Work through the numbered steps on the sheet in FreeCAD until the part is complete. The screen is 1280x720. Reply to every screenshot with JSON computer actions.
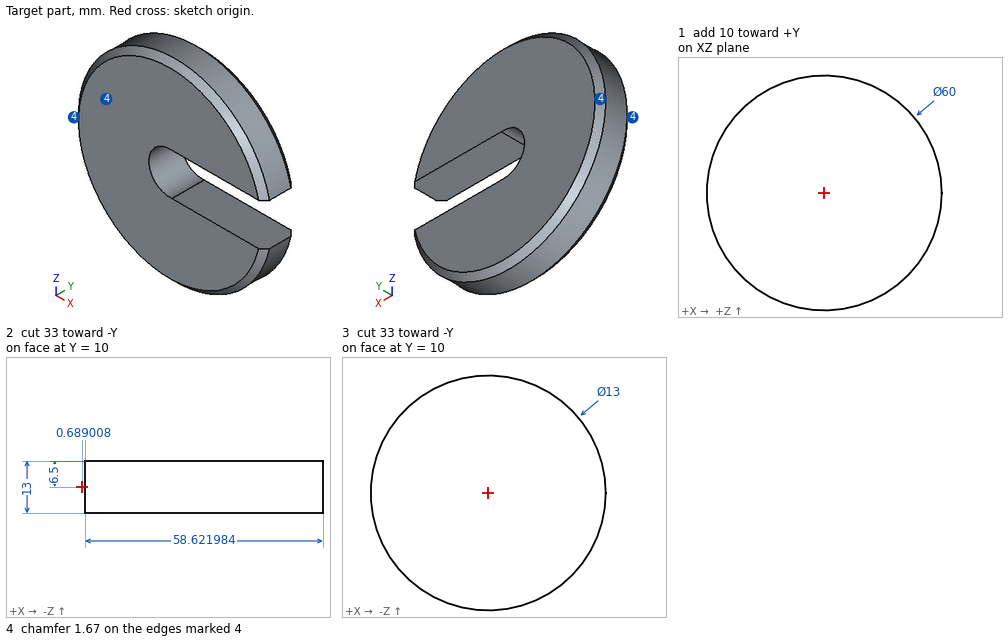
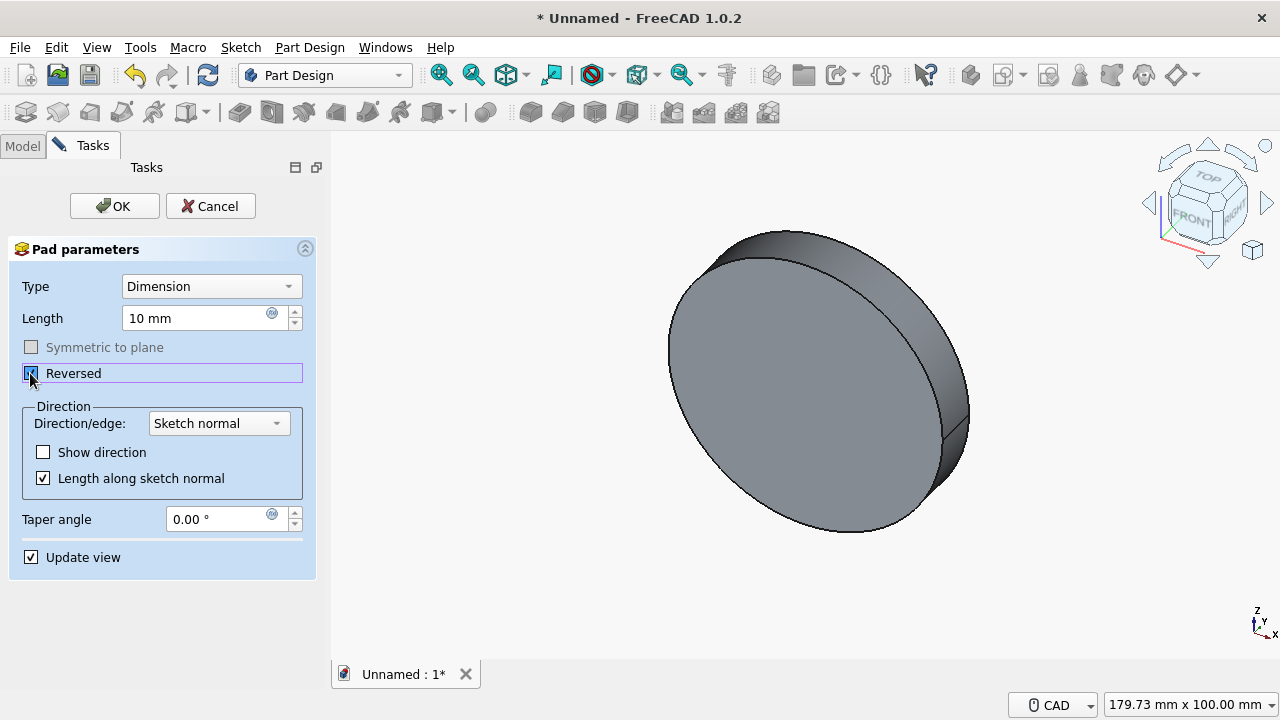
{"action": "left_click", "coordinate": [115, 206]}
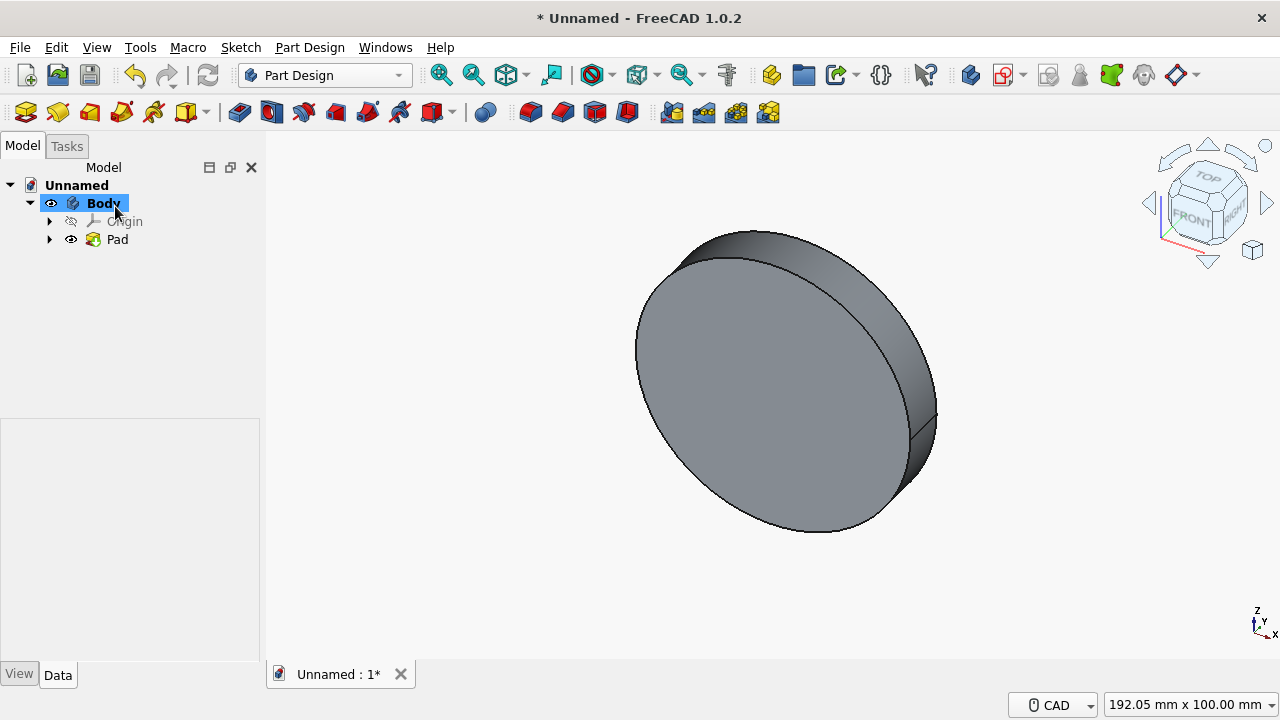
{"action": "key", "text": "4"}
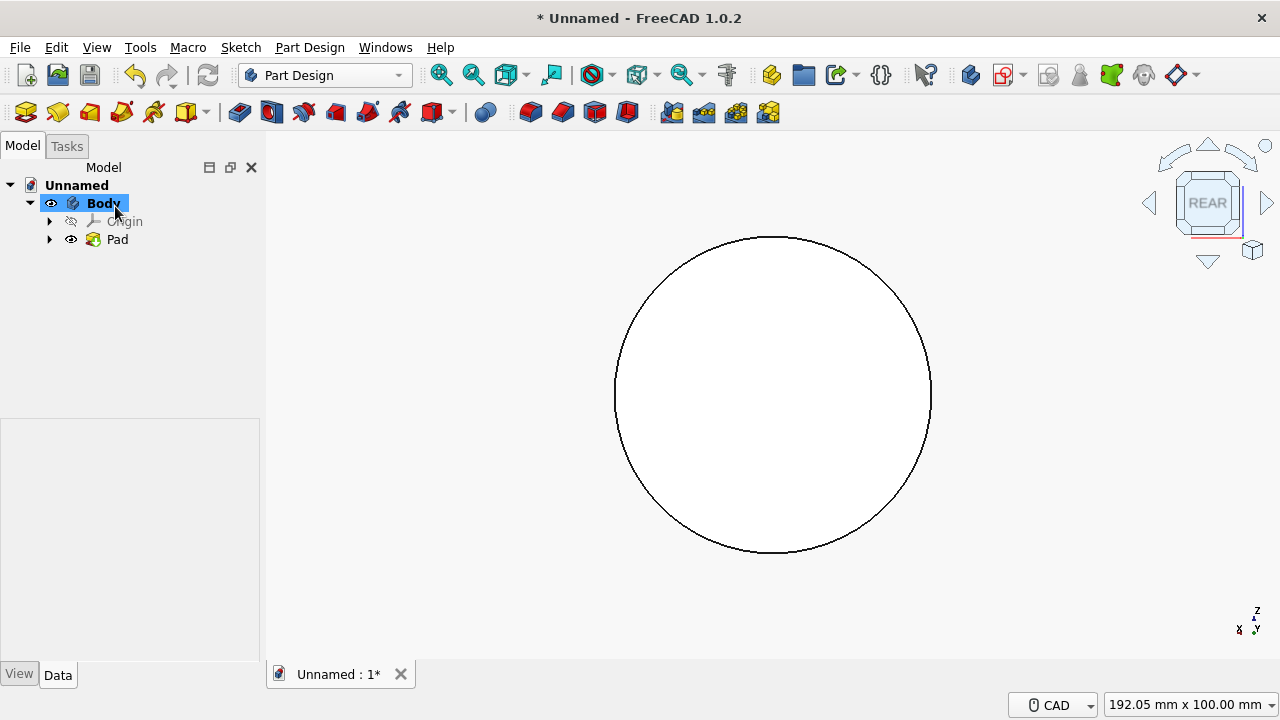
{"action": "left_click", "coordinate": [773, 394]}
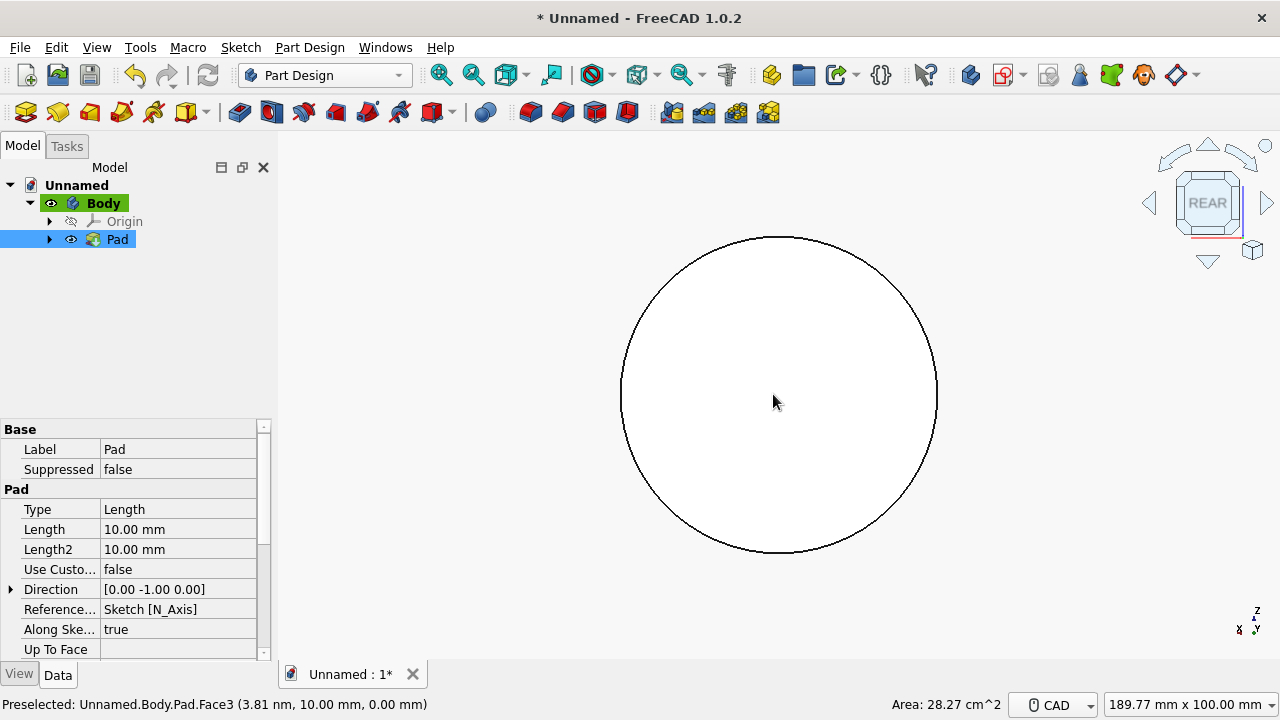
{"action": "left_click", "coordinate": [1004, 76]}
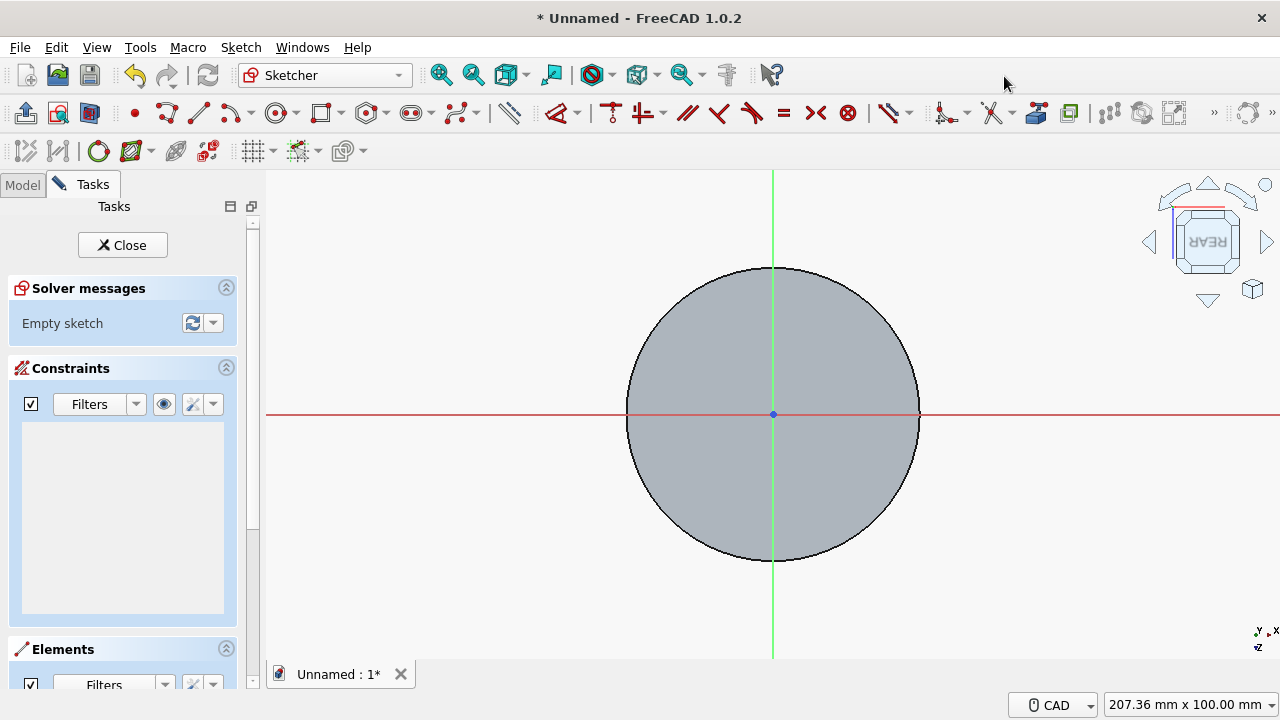
{"action": "scroll", "coordinate": [1115, 415], "scroll_direction": "up", "scroll_amount": 3}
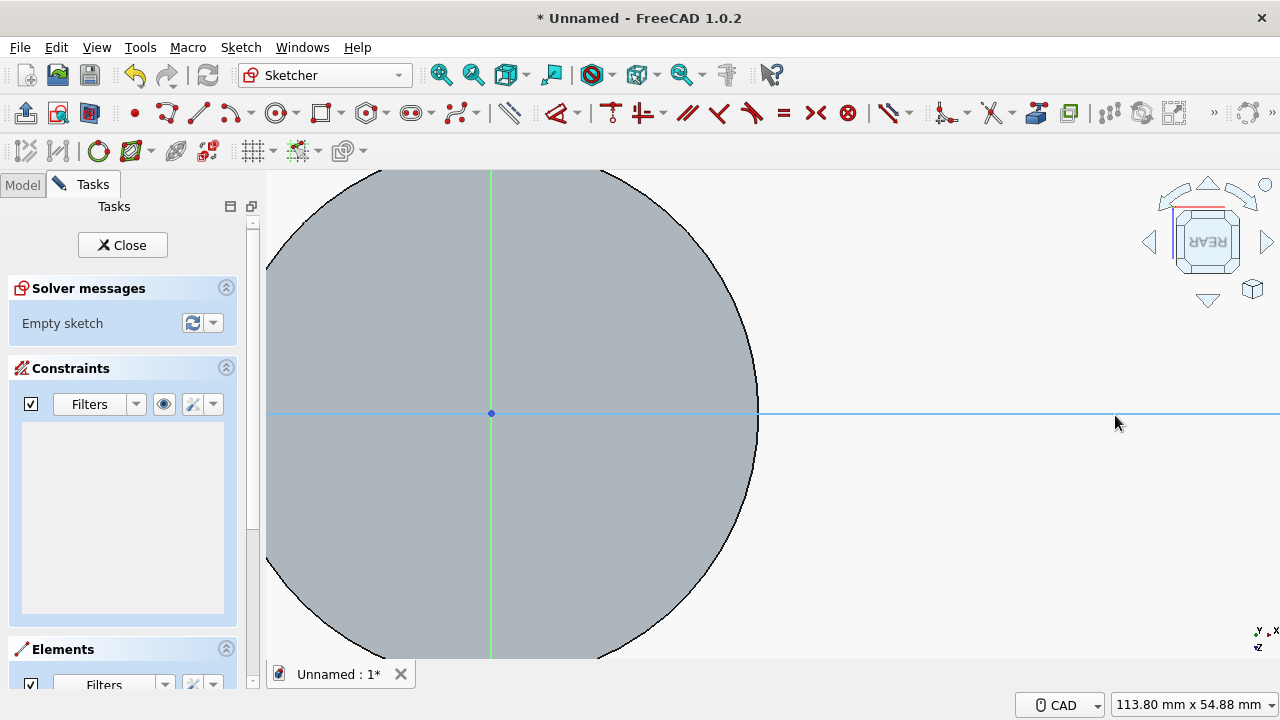
{"action": "key", "text": "g r"}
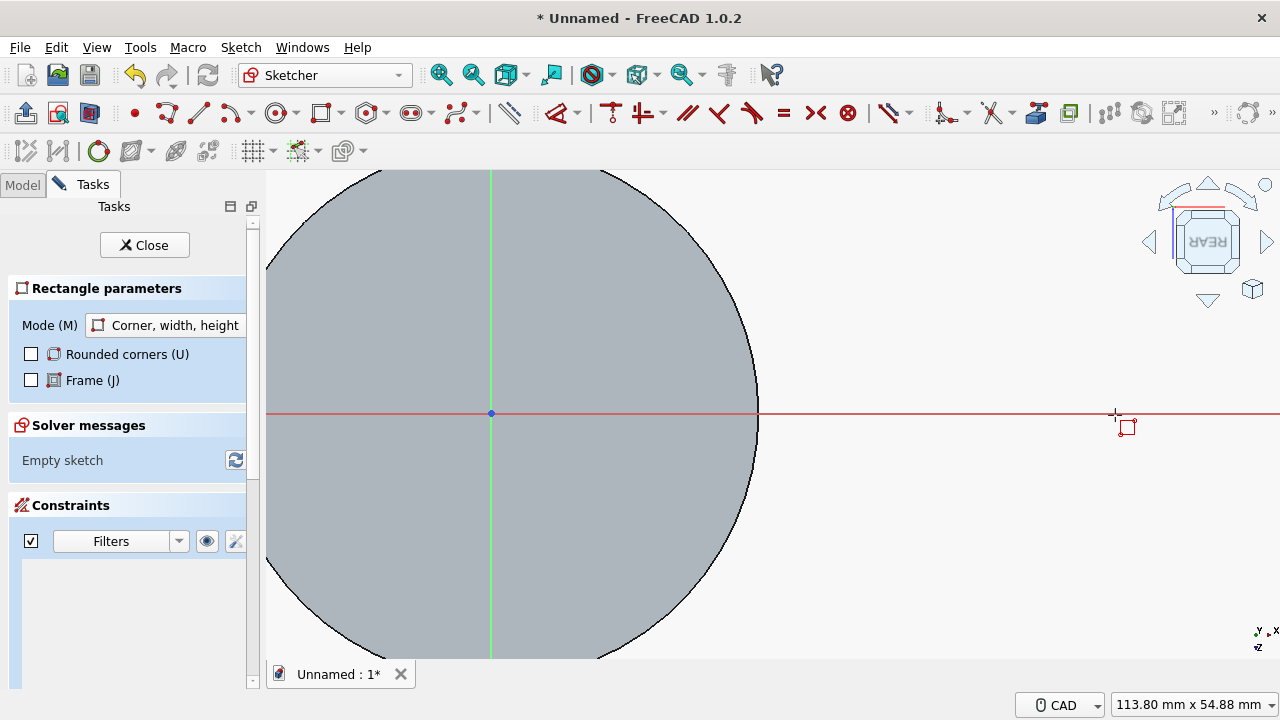
{"action": "scroll", "coordinate": [497, 356], "scroll_direction": "up", "scroll_amount": 5}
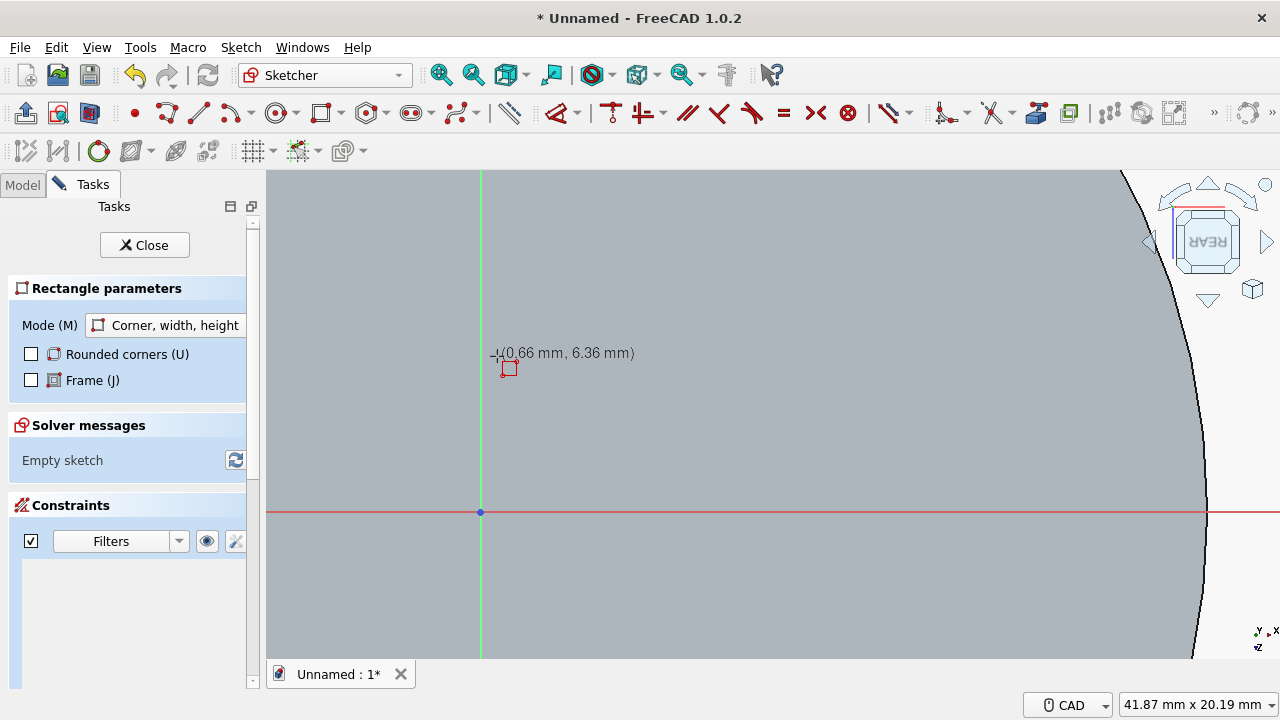
{"action": "left_click", "coordinate": [497, 355]}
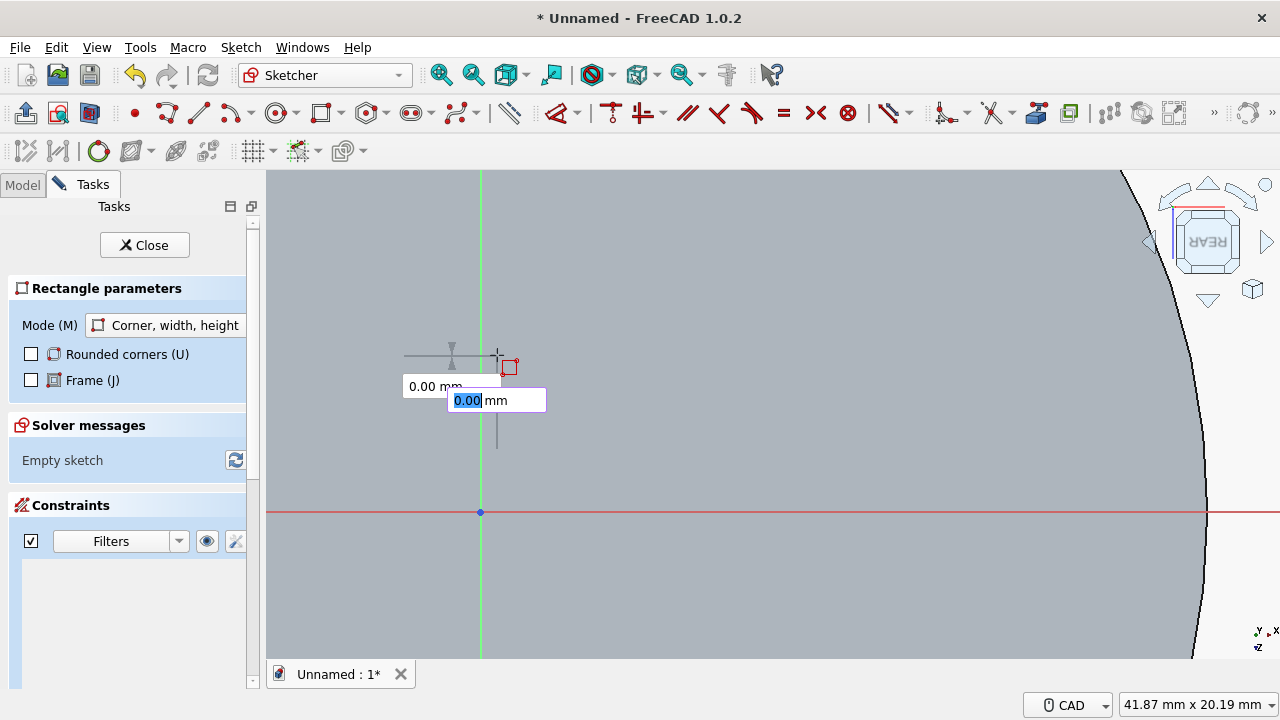
{"action": "scroll", "coordinate": [417, 358], "scroll_direction": "down", "scroll_amount": 5}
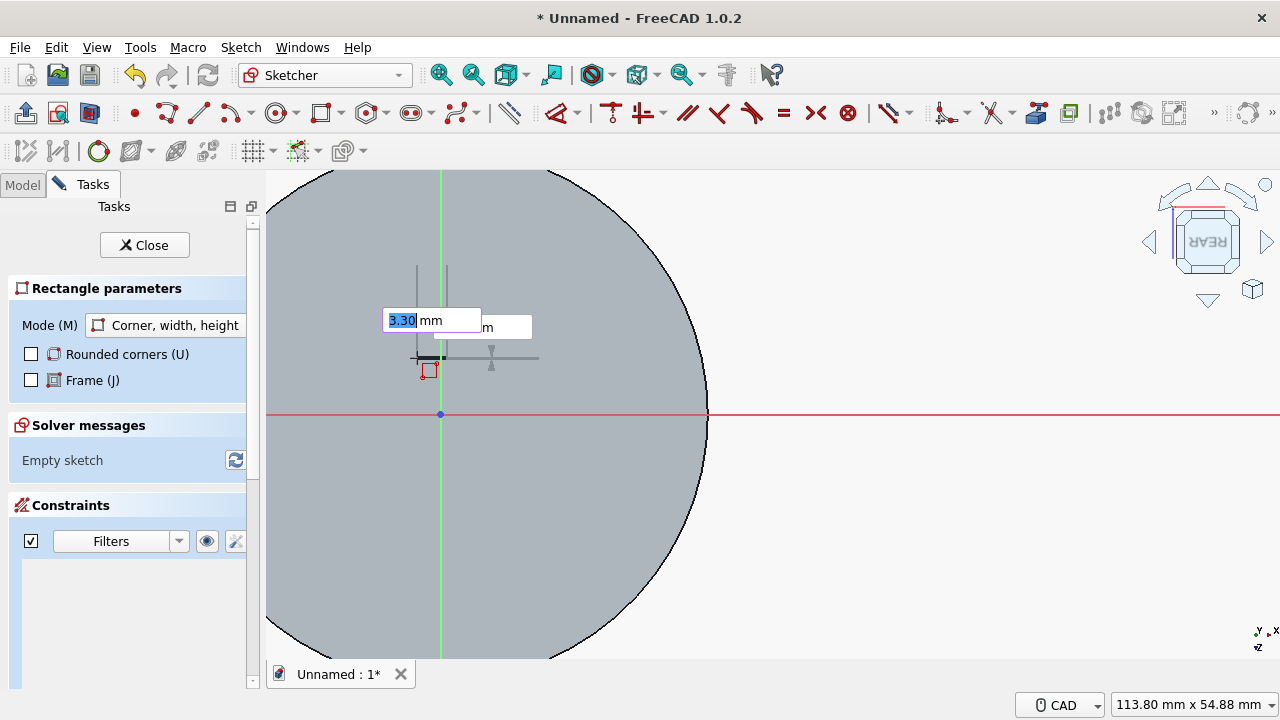
{"action": "left_click", "coordinate": [969, 473]}
{"action": "key", "text": "Escape"}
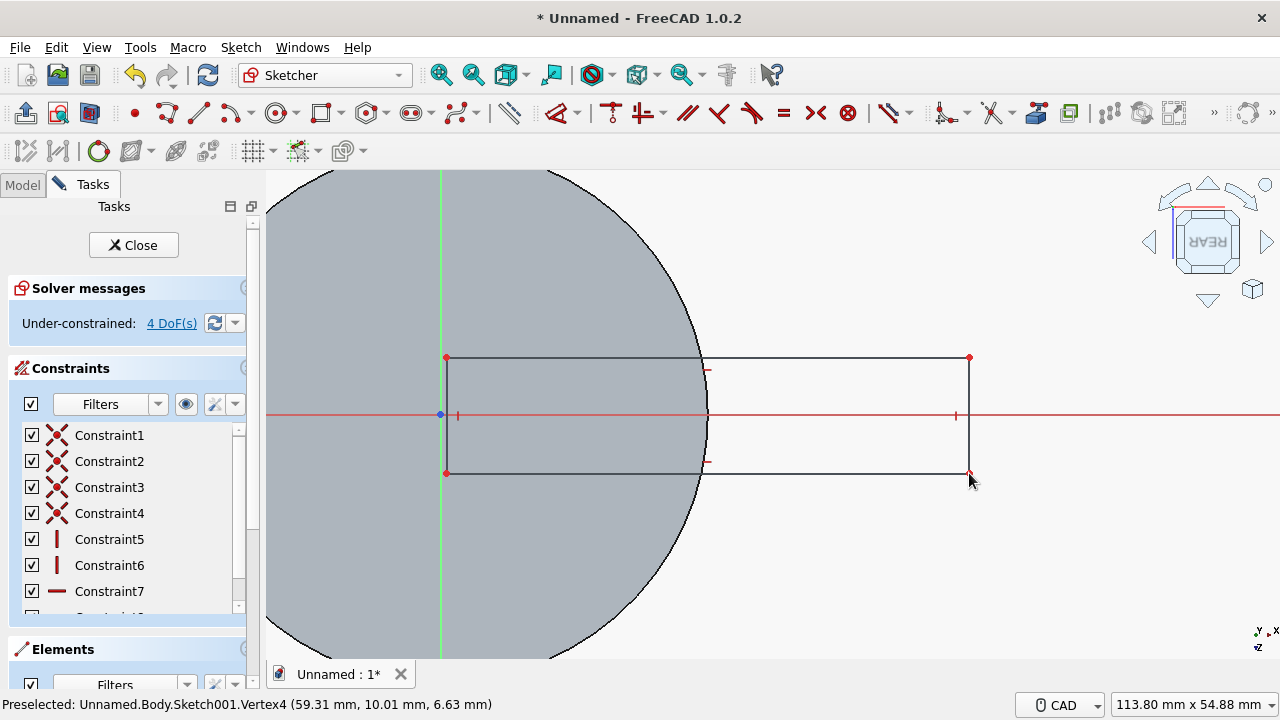
{"action": "key", "text": "d"}